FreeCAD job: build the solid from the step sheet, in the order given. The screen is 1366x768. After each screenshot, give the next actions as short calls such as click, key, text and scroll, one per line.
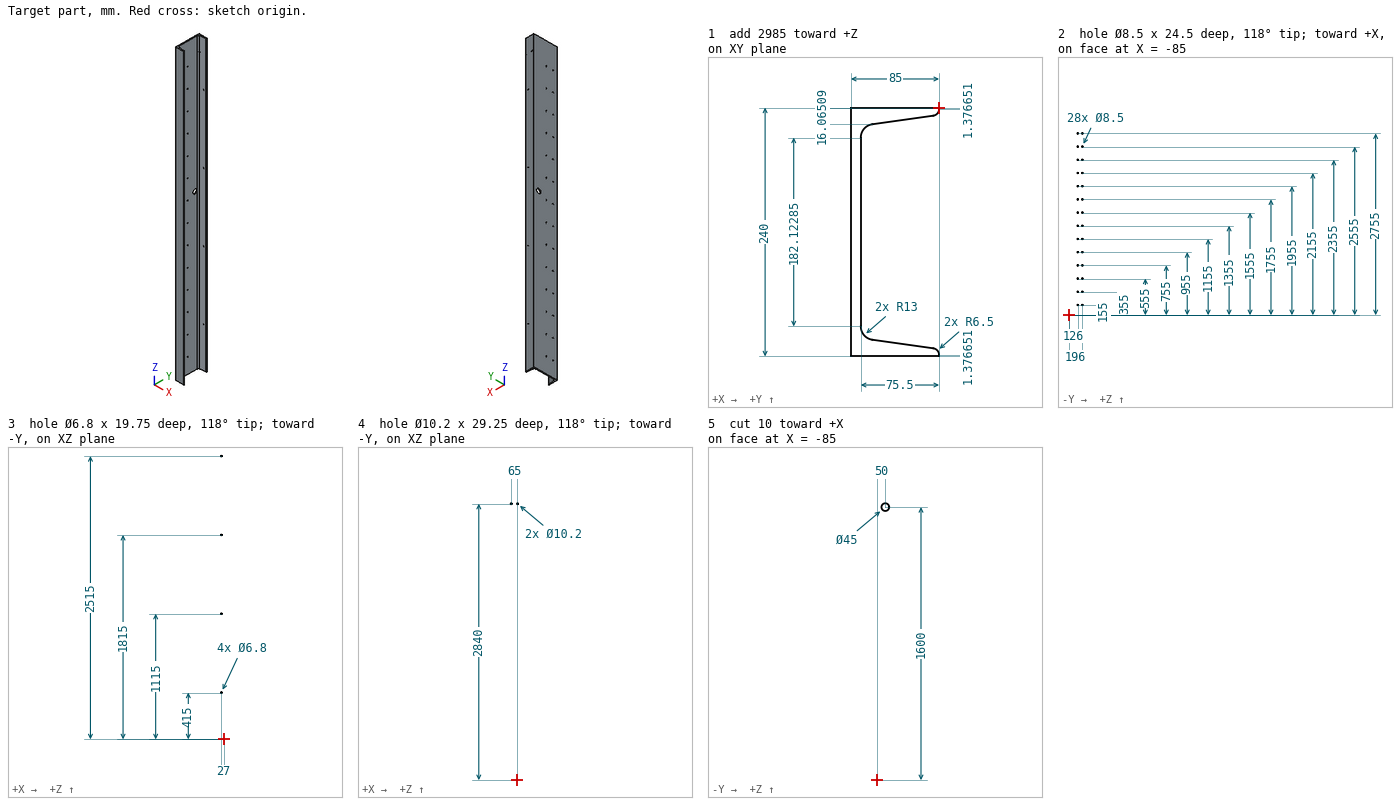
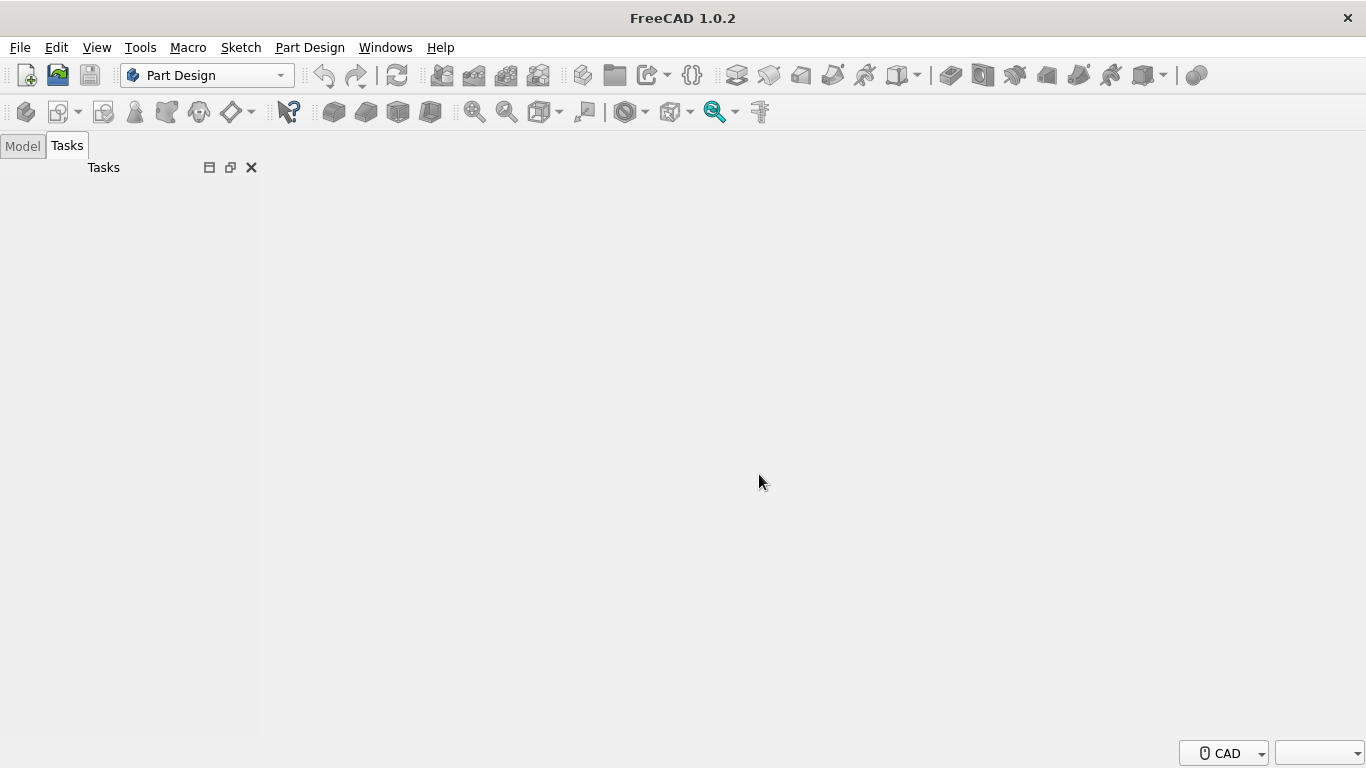
click(26, 76)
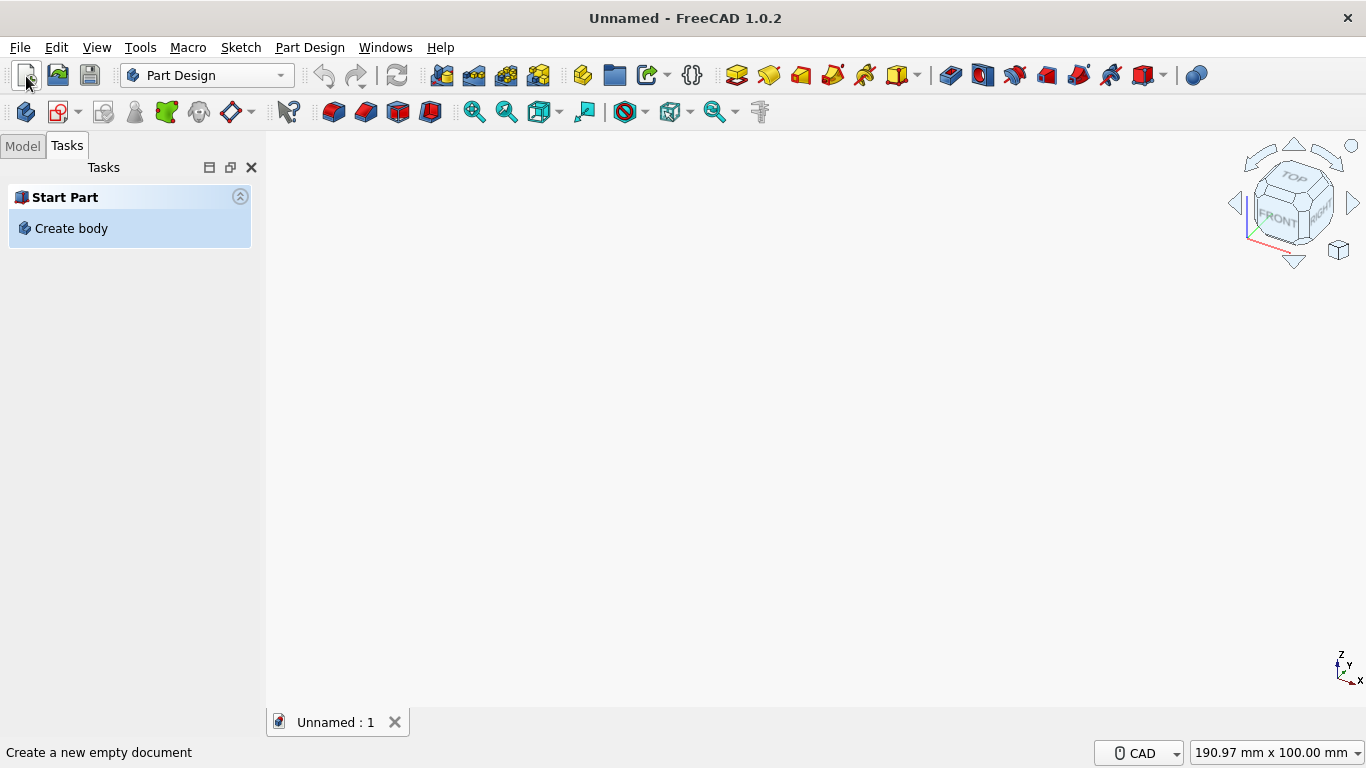
click(58, 112)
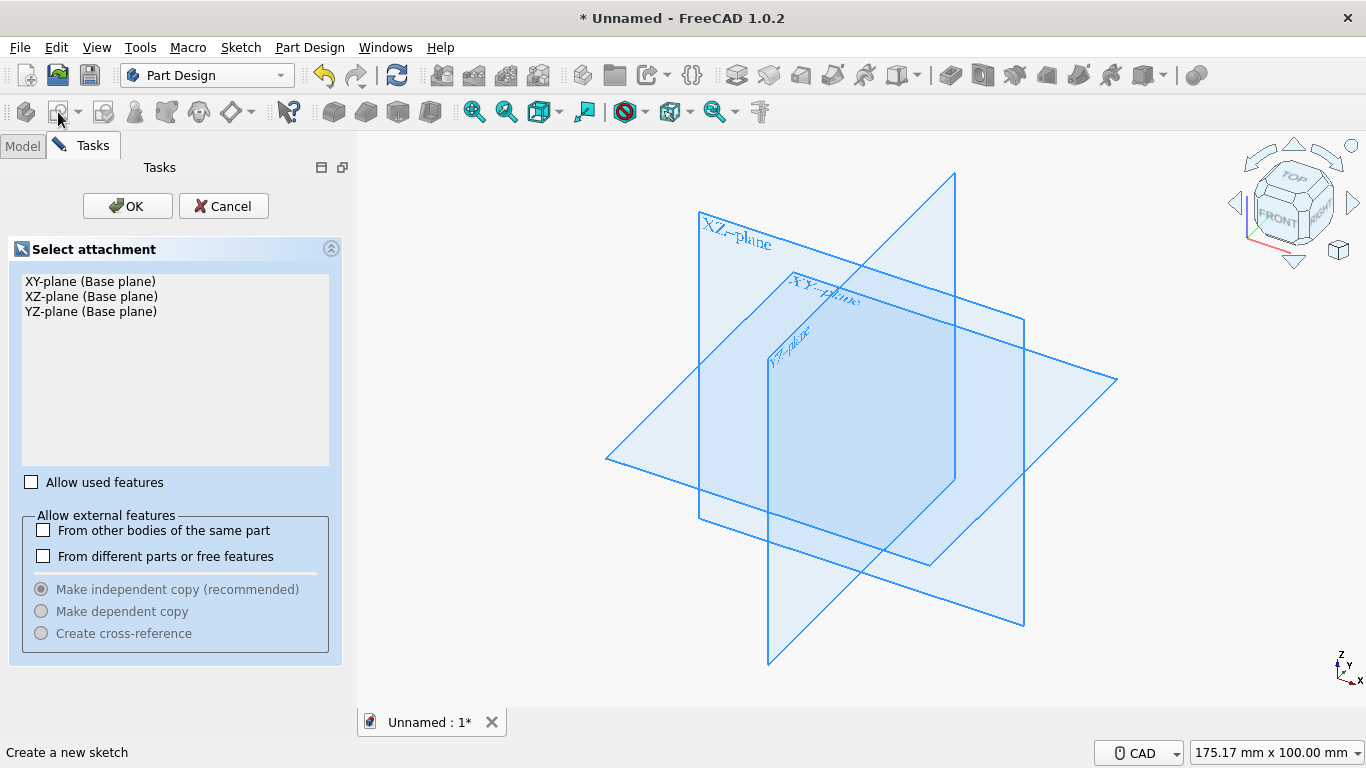
click(82, 282)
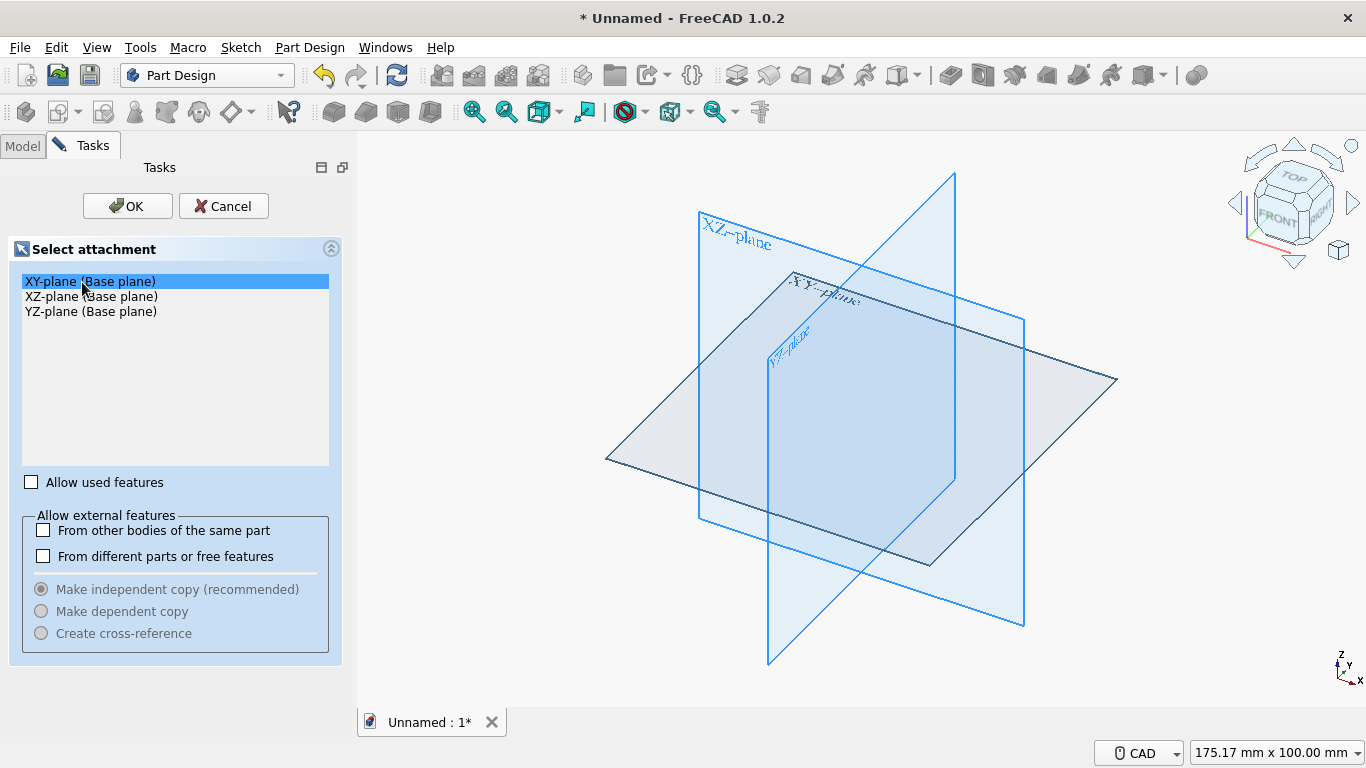
click(128, 206)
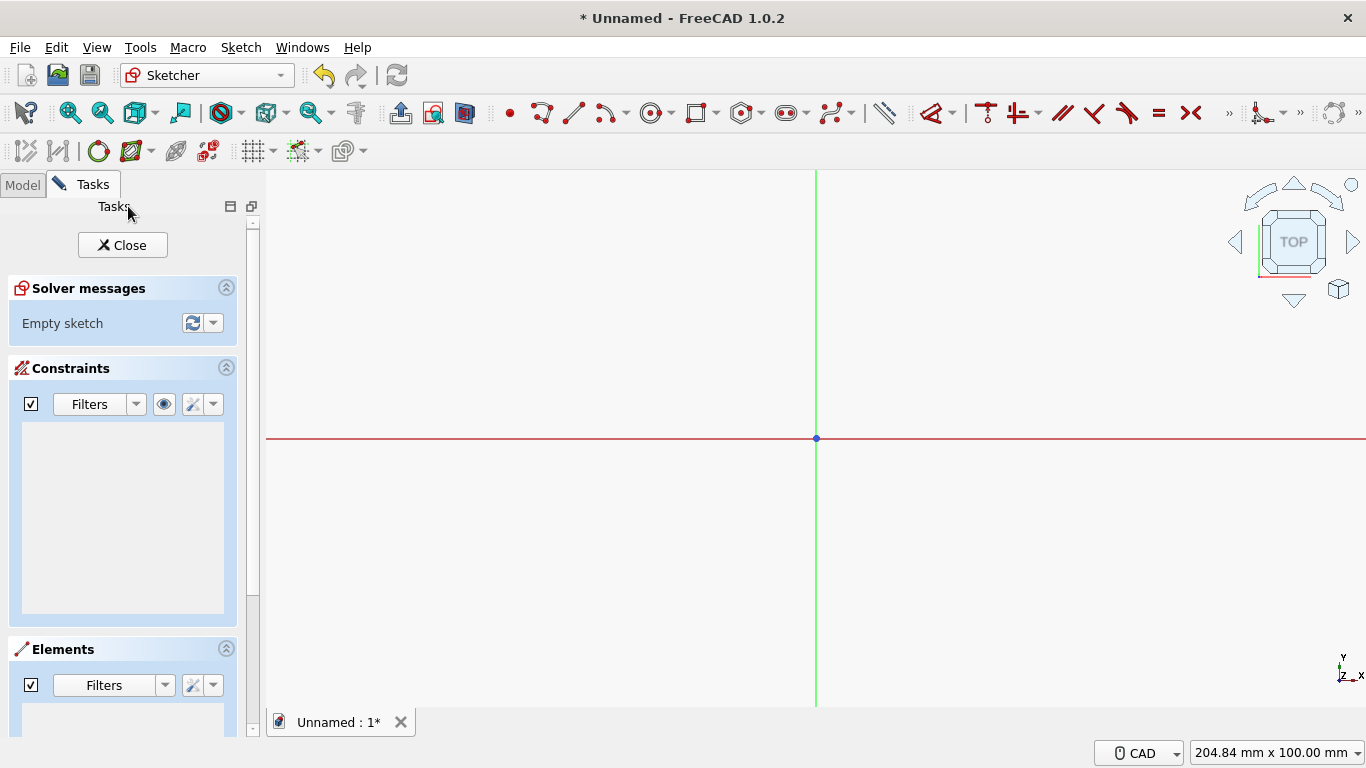
scroll(800, 228, down, 7)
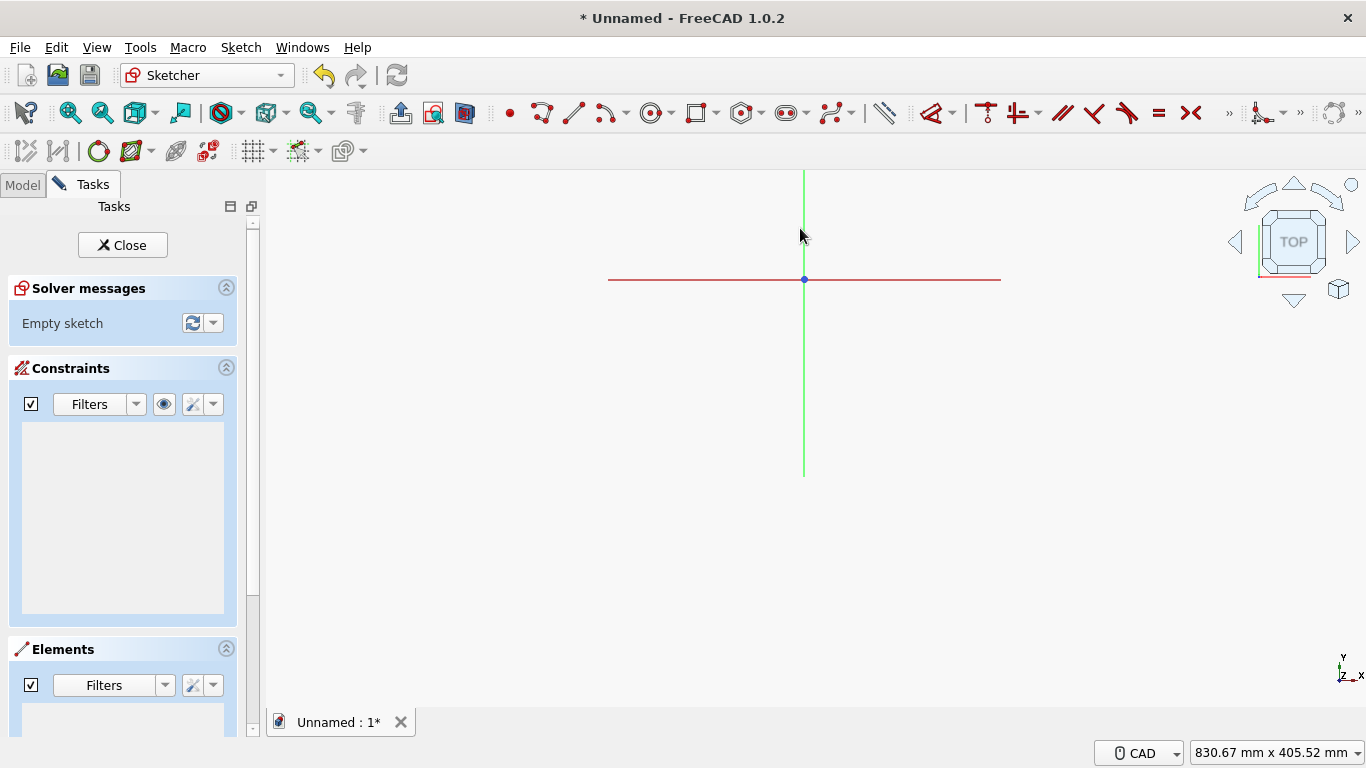
click(574, 114)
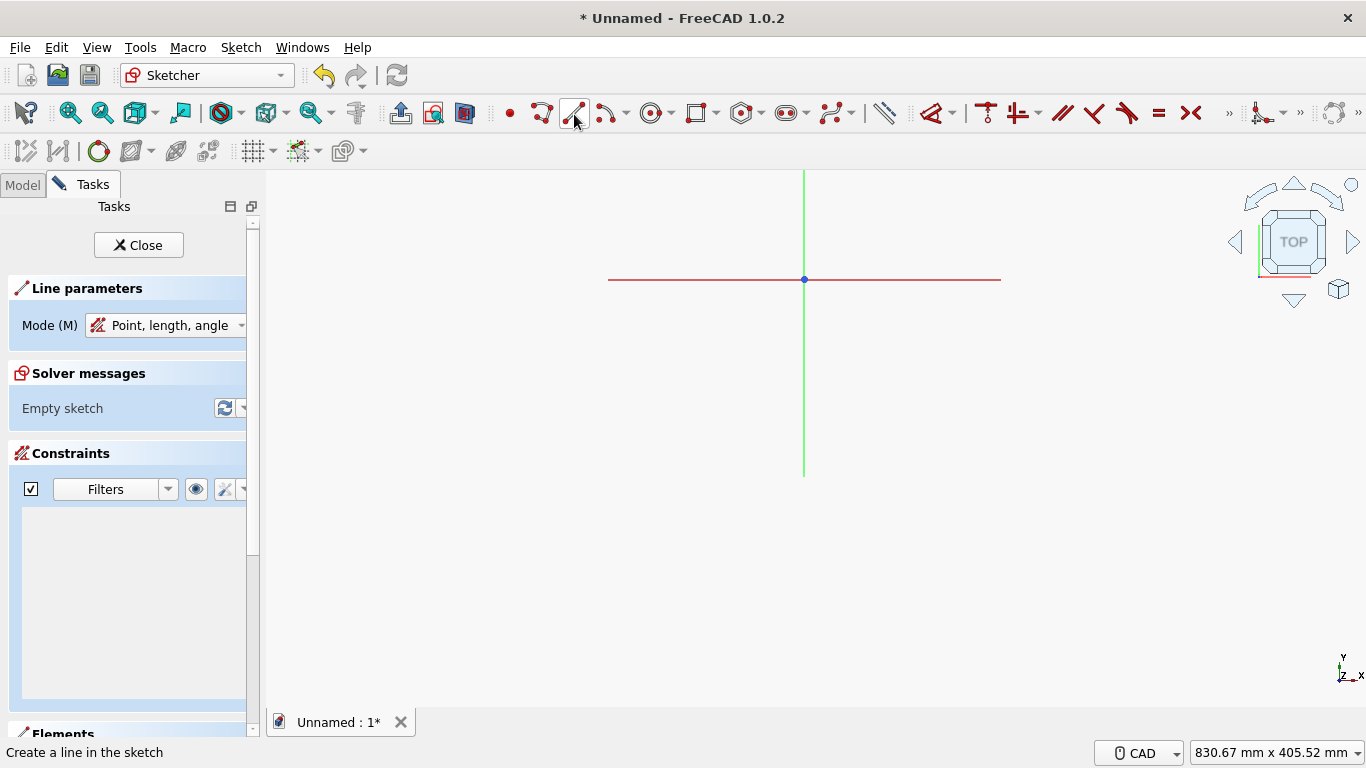
scroll(797, 587, up, 4)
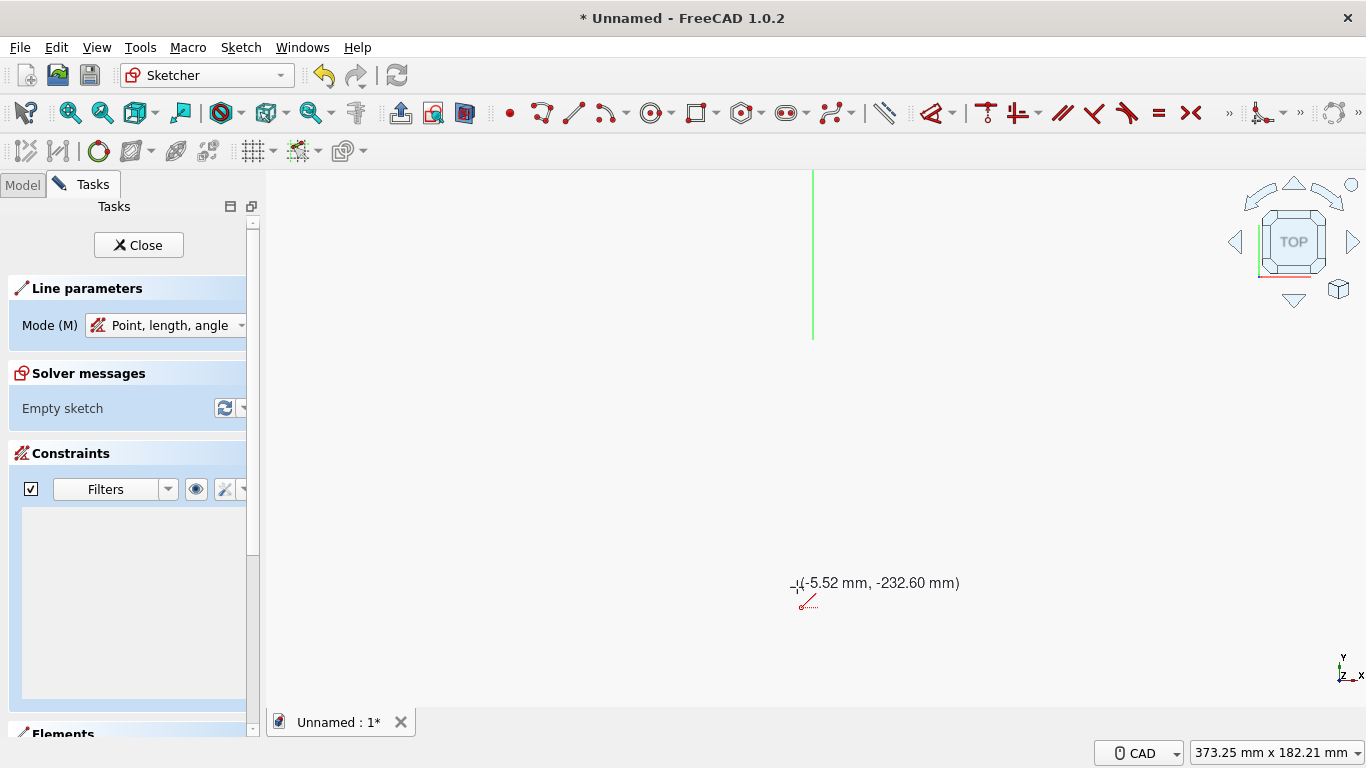
click(796, 587)
click(623, 563)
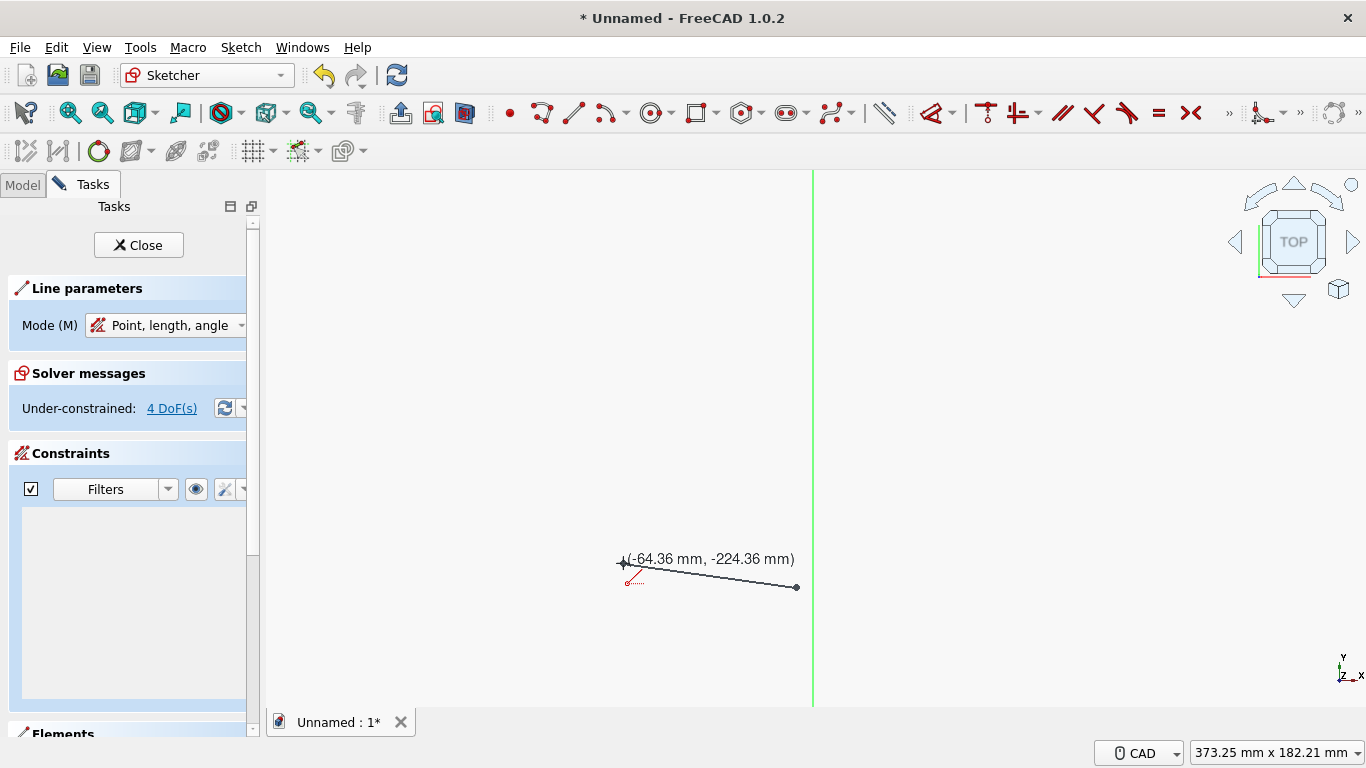
click(590, 525)